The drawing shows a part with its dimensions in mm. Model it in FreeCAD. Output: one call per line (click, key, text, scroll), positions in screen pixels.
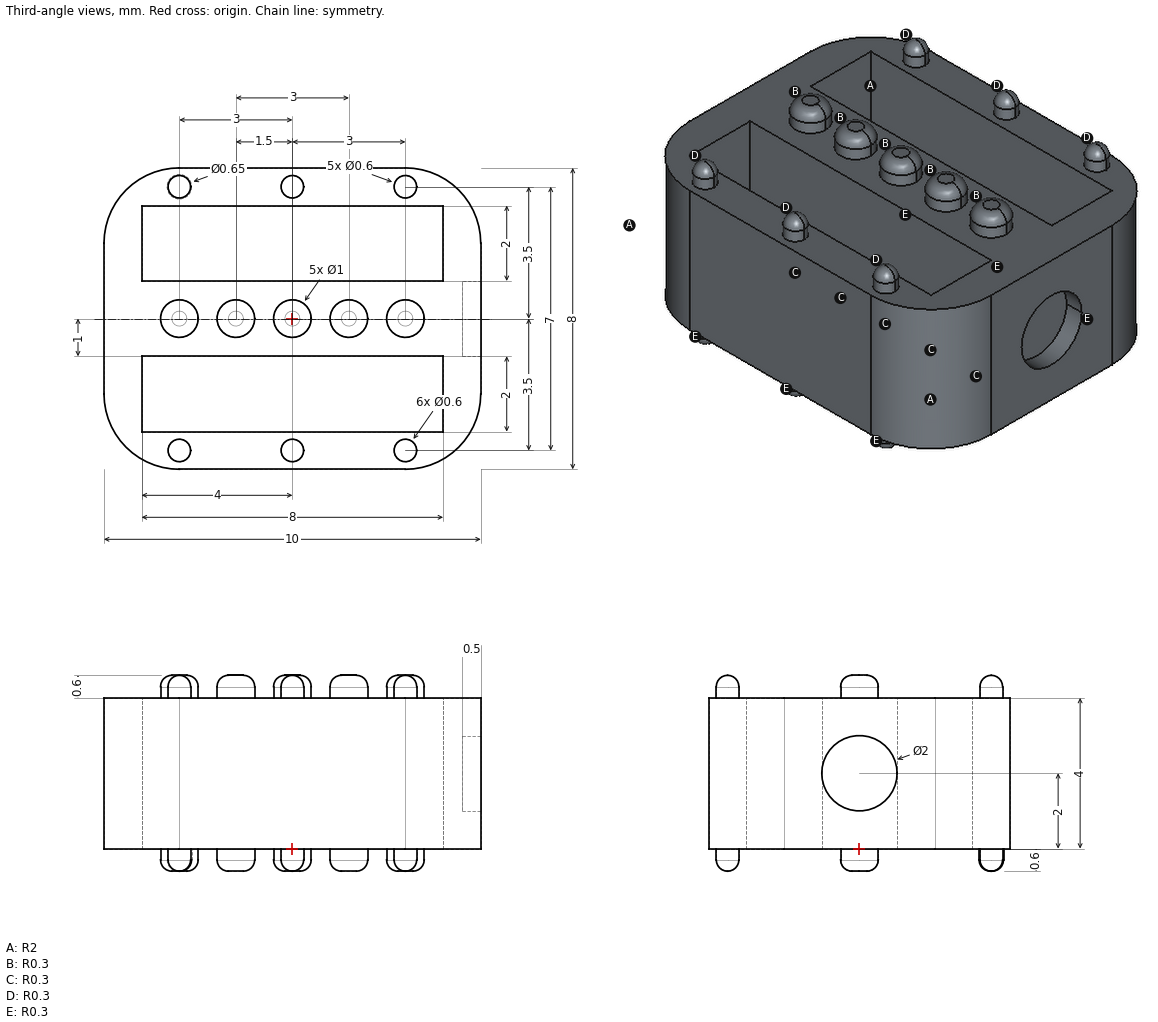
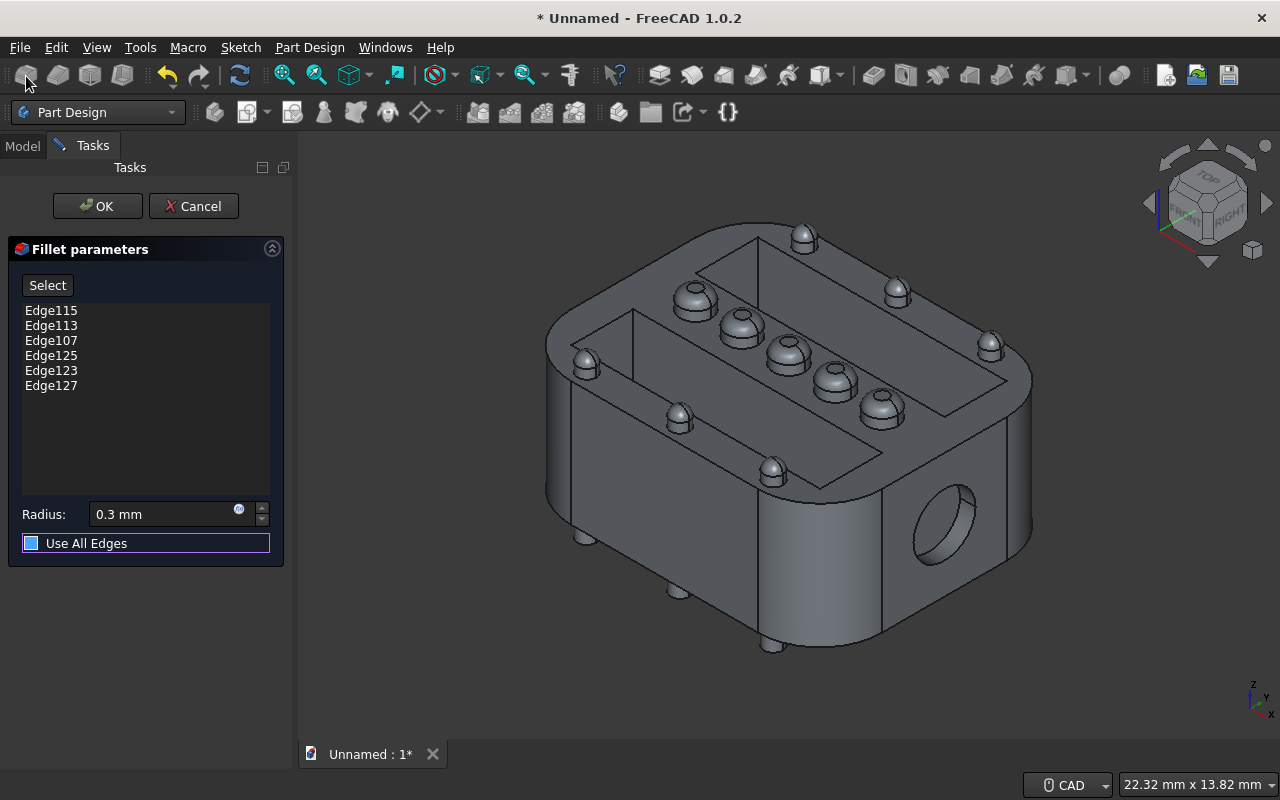
click(98, 206)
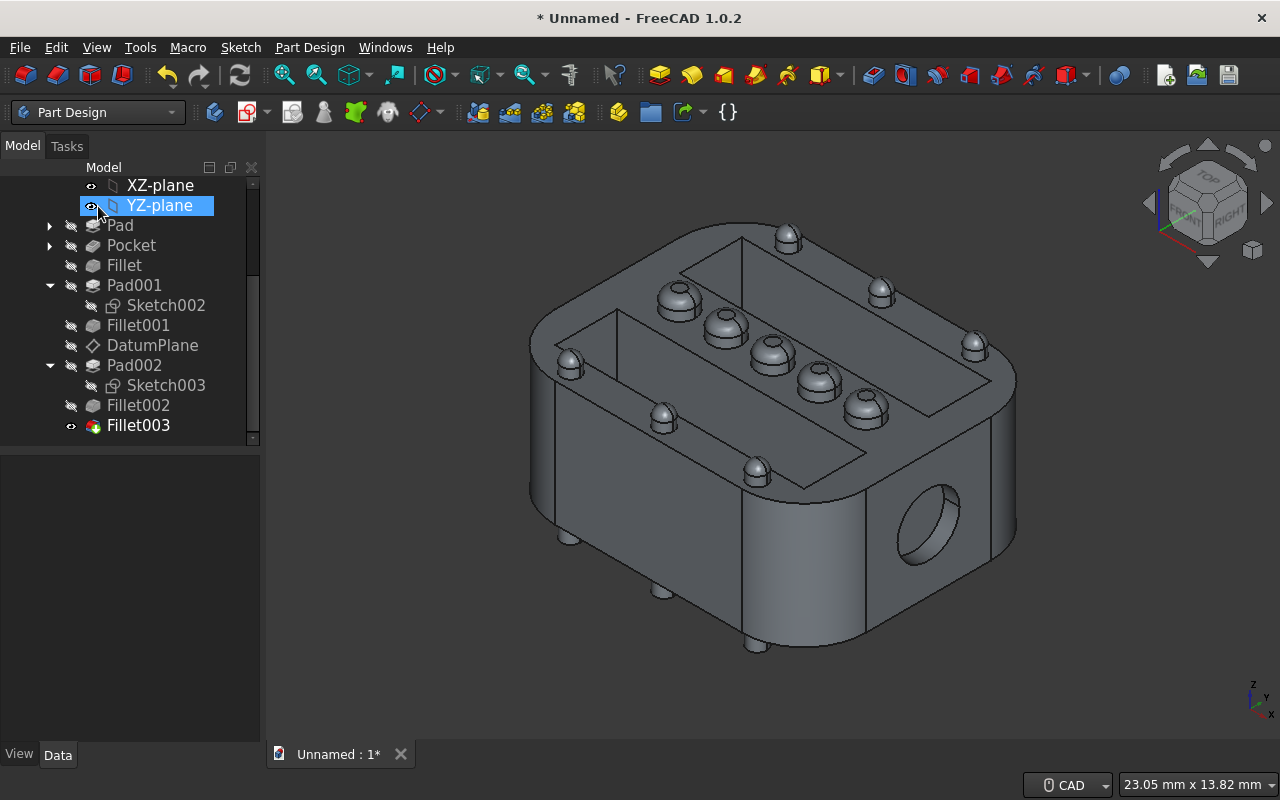
click(746, 648)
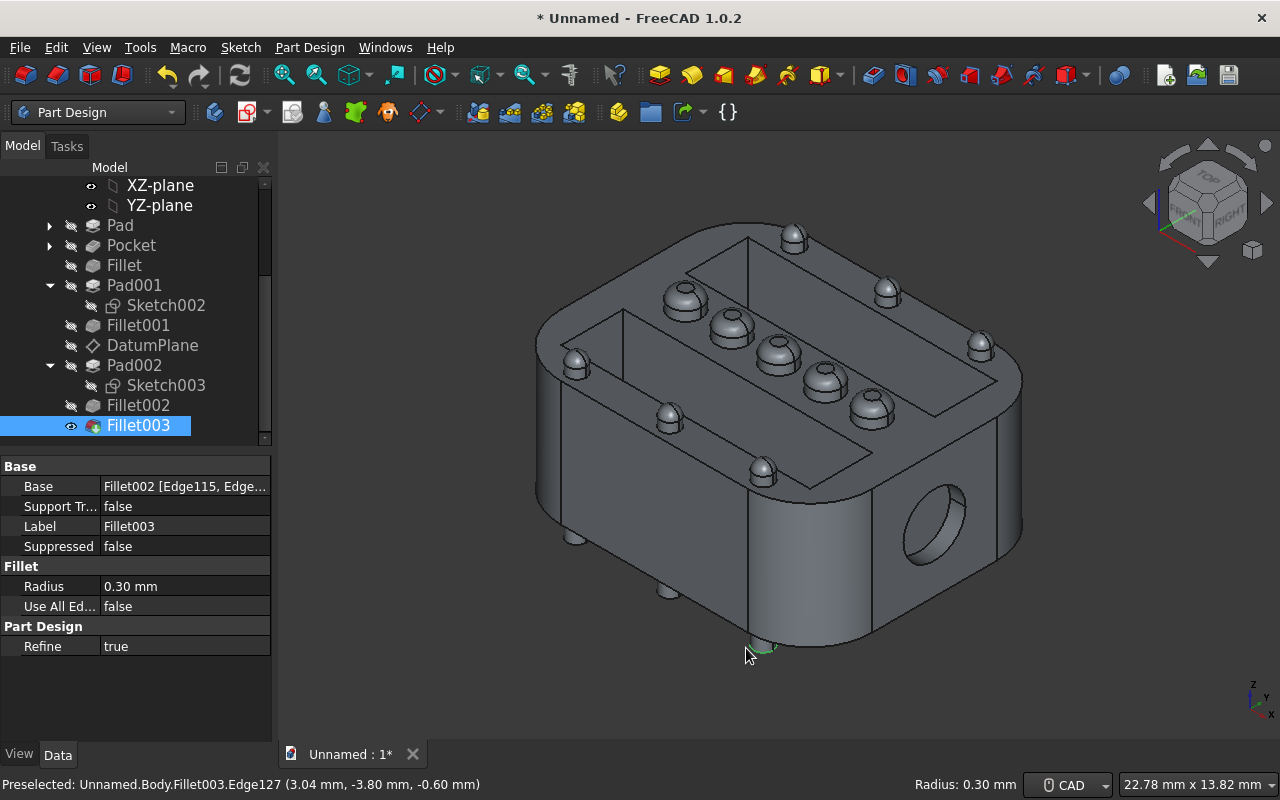
click(658, 594, ctrl)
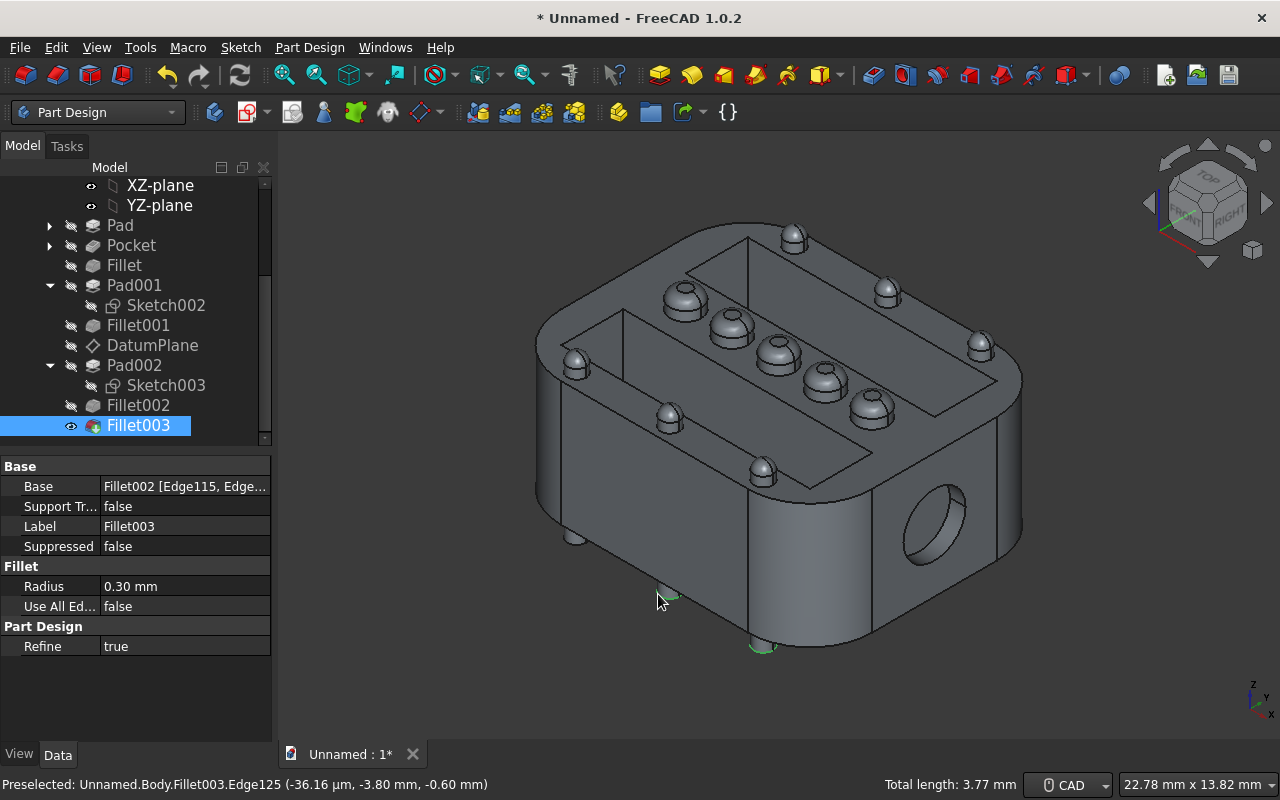
click(565, 540, ctrl)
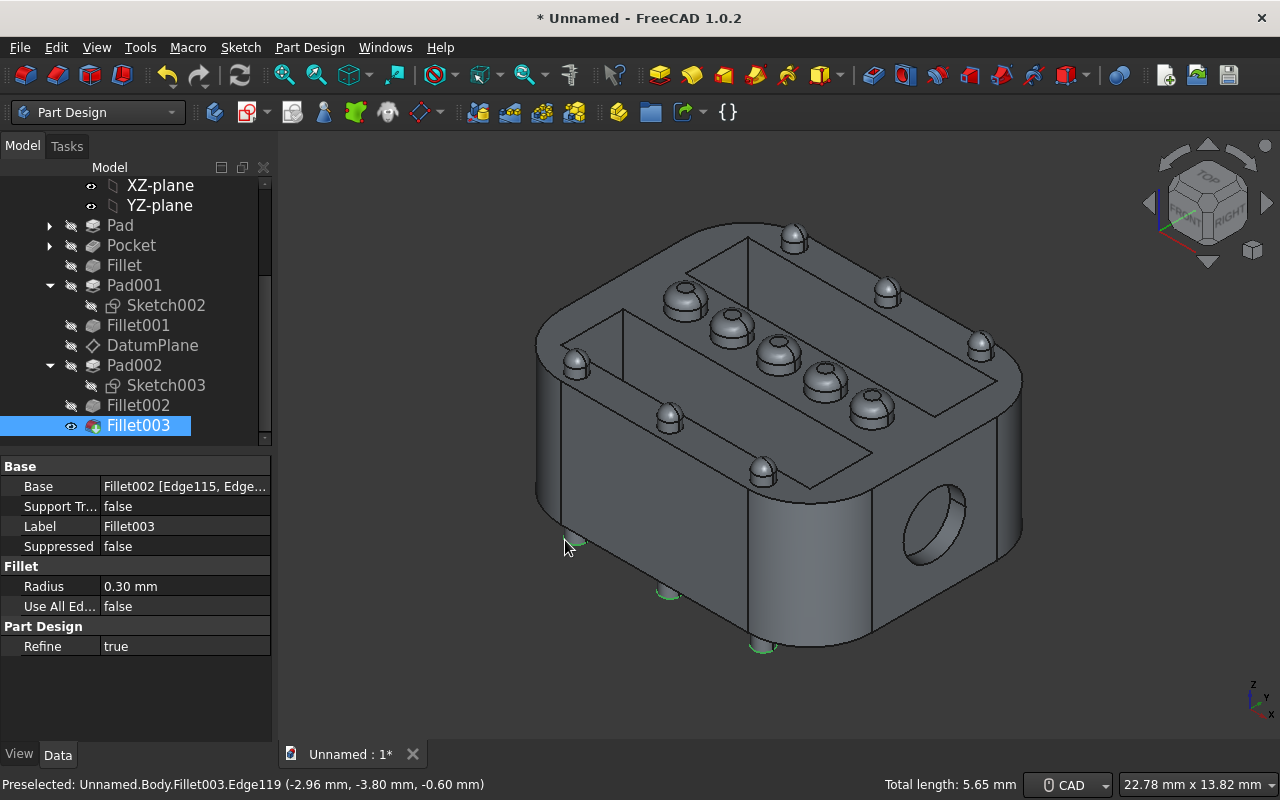
key(2)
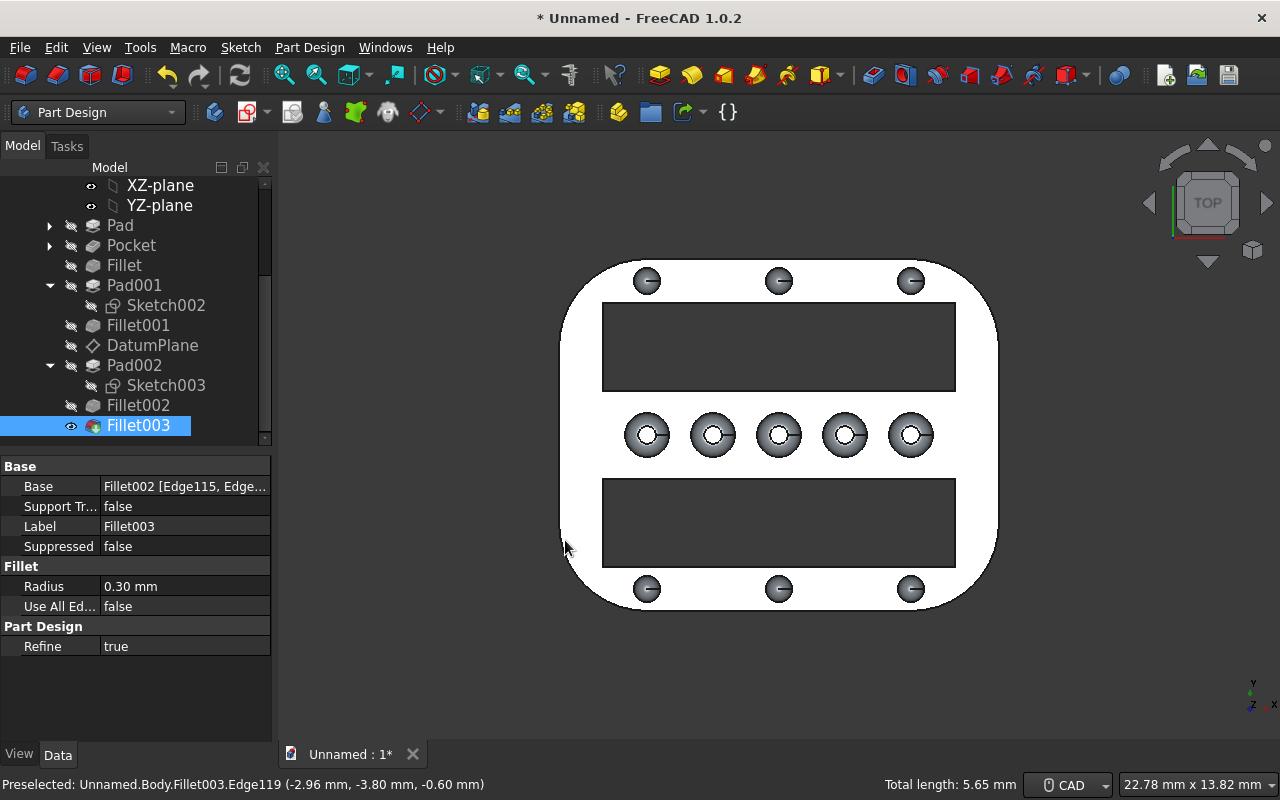
key(0)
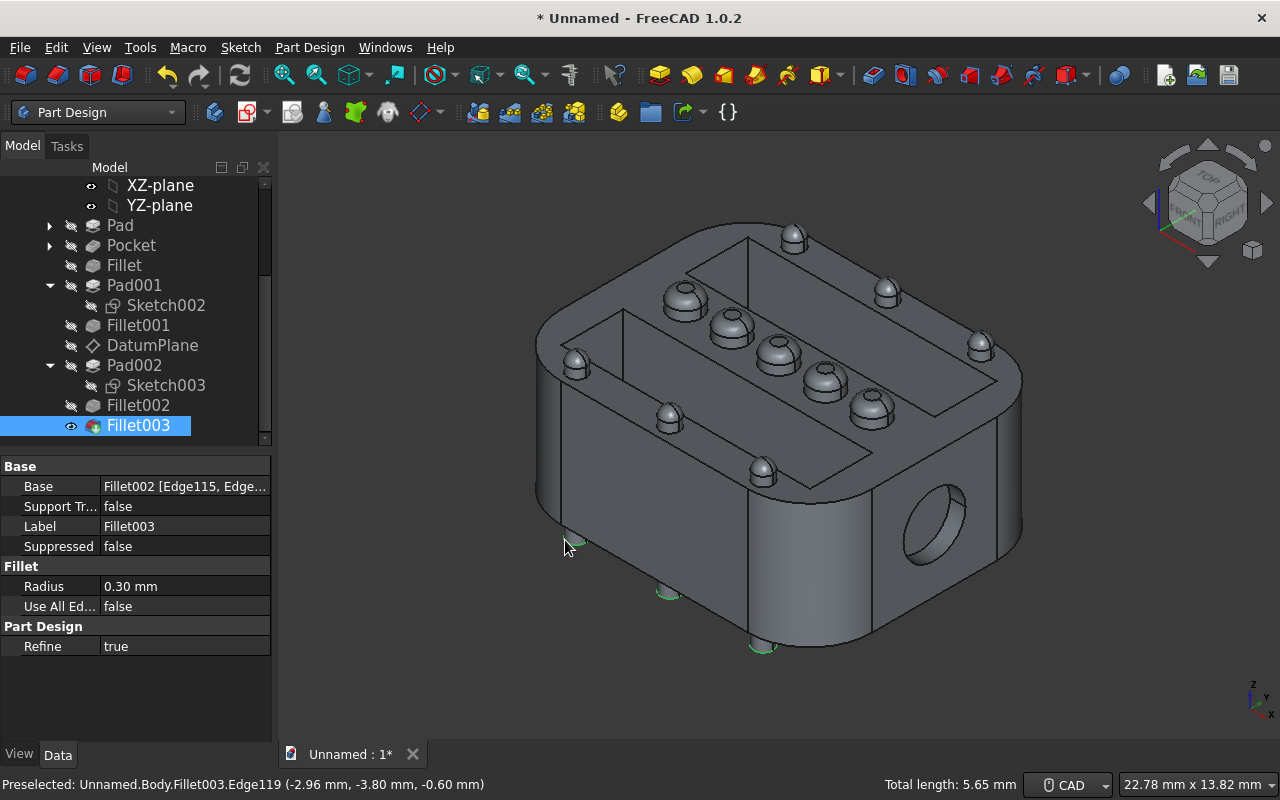
key(1)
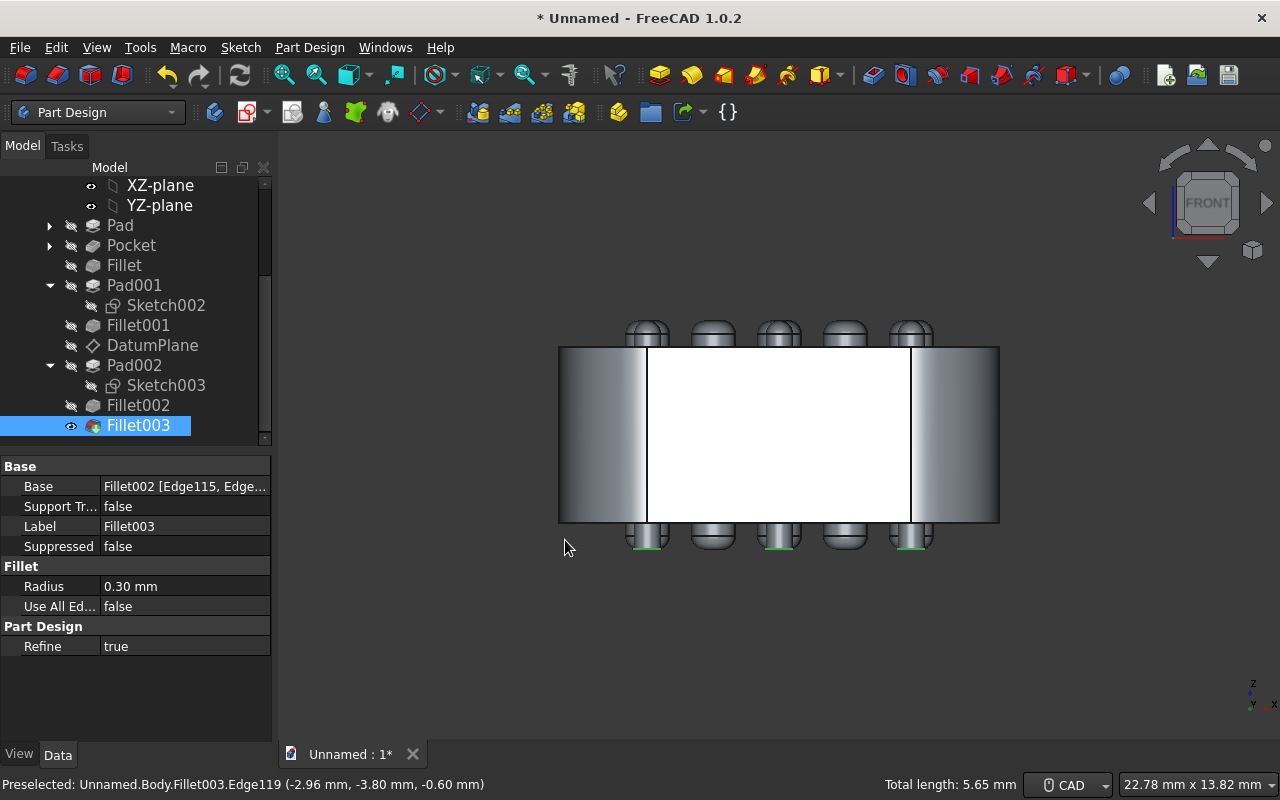
click(286, 76)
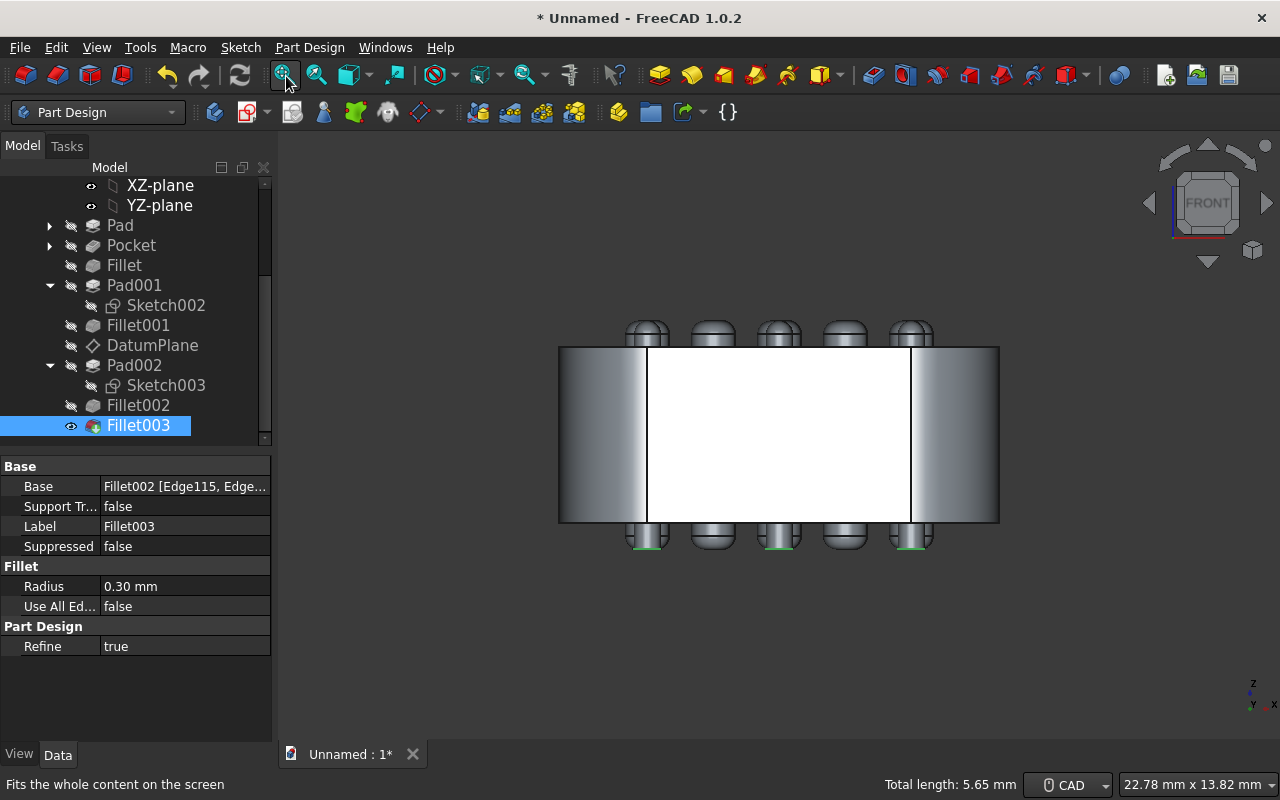
key(3)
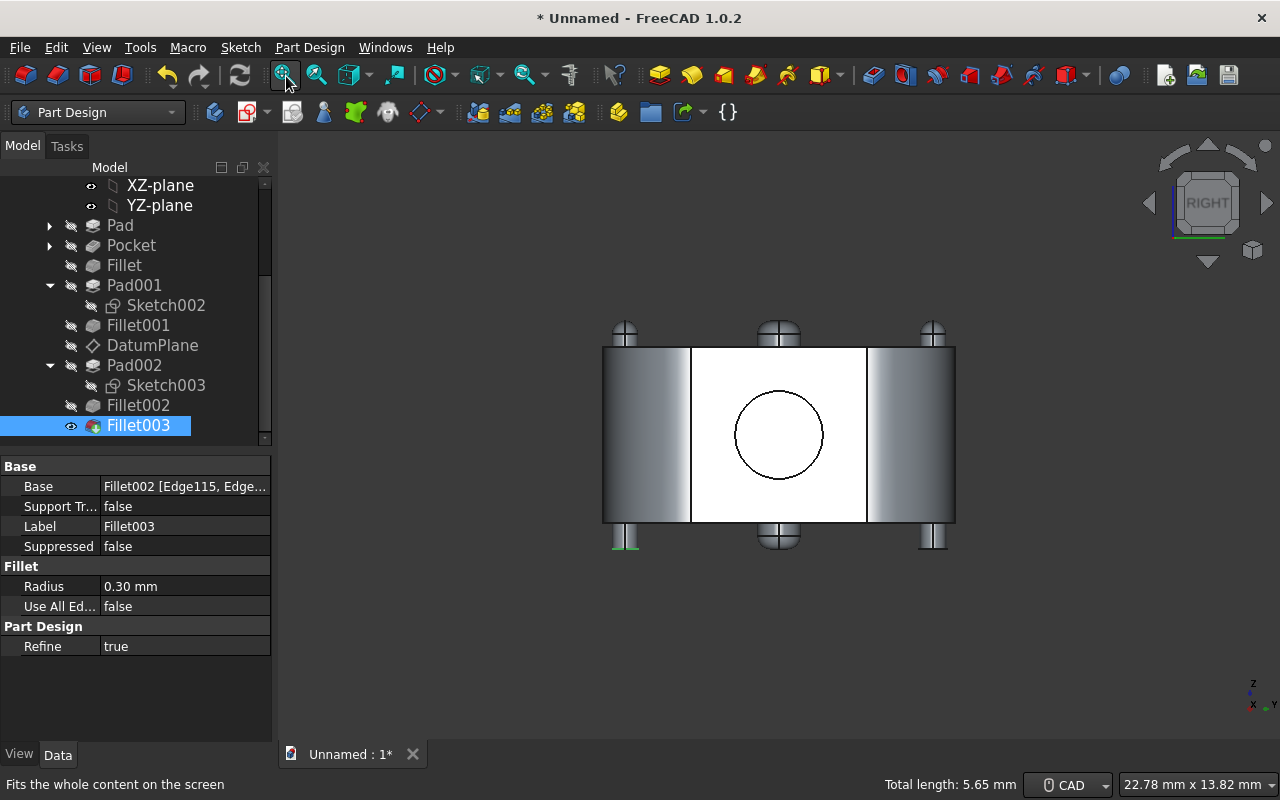
click(286, 76)